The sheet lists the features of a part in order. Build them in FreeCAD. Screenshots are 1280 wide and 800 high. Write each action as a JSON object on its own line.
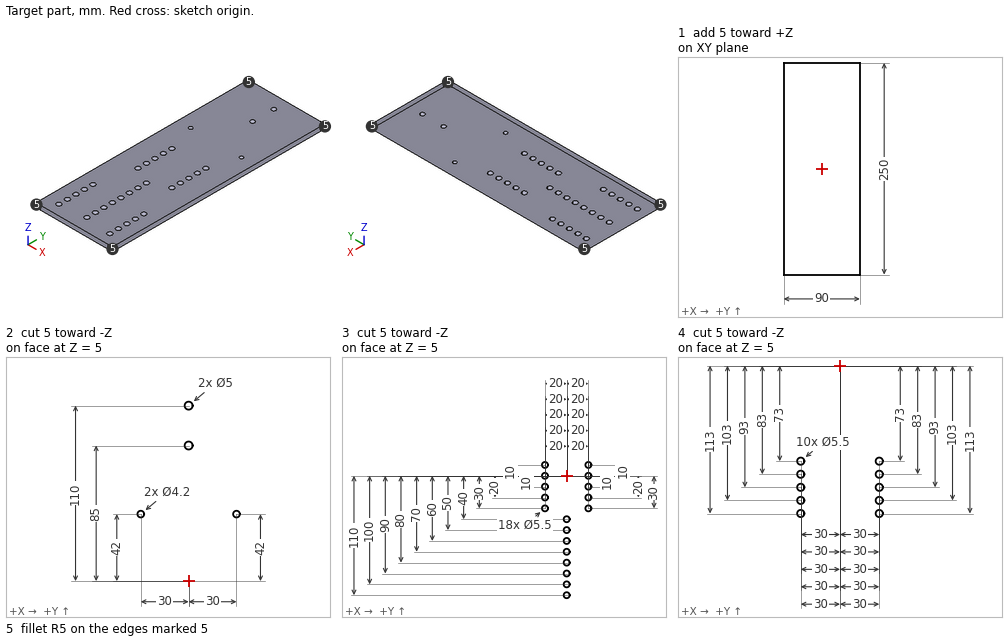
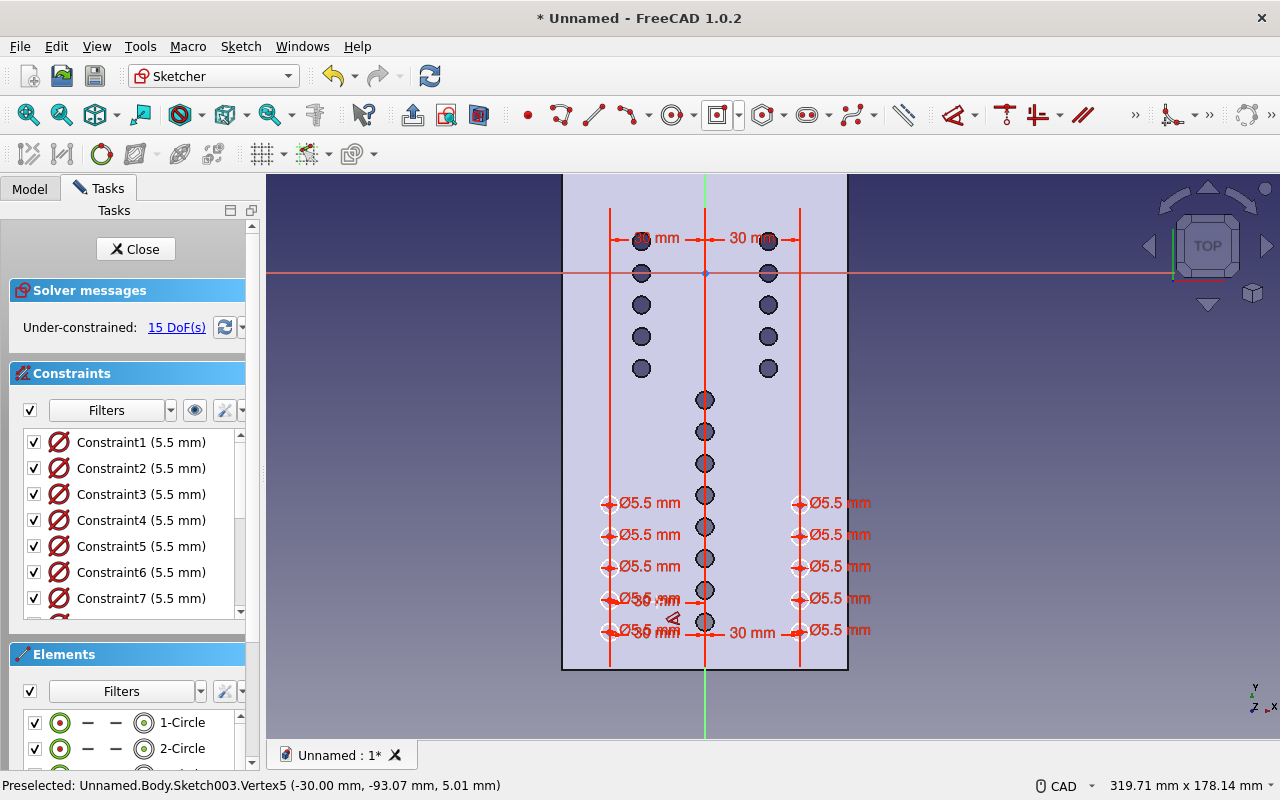
{"action": "left_click", "coordinate": [610, 568]}
{"action": "left_click", "coordinate": [576, 421]}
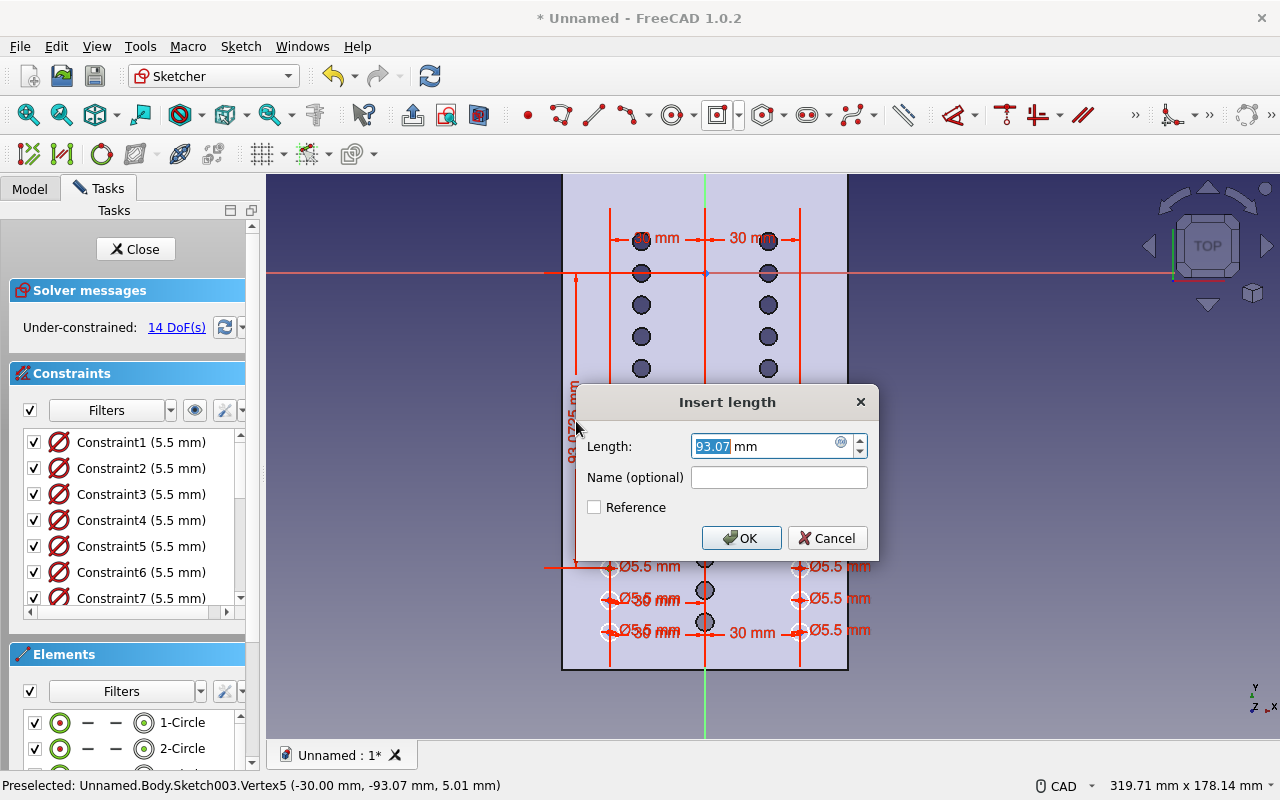
{"action": "type", "text": "93"}
{"action": "key", "text": "Return"}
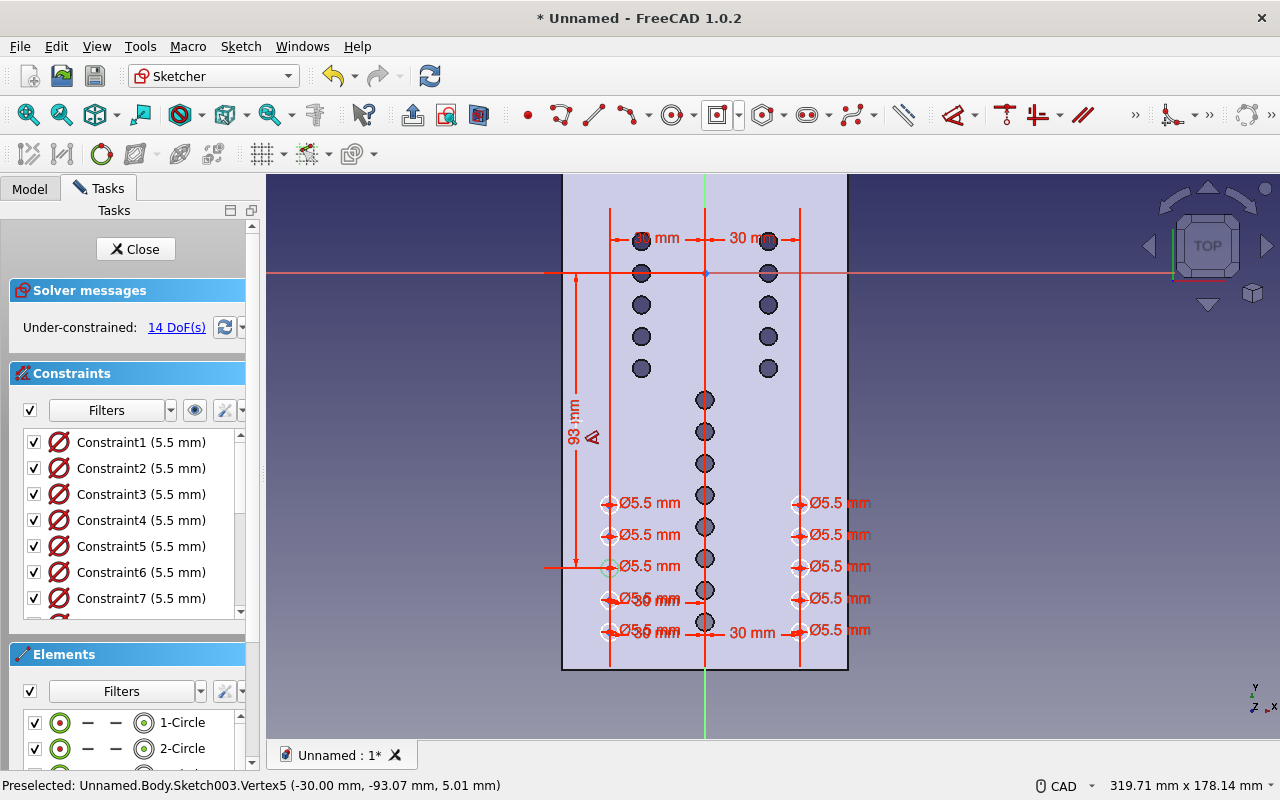
{"action": "left_click", "coordinate": [800, 568]}
{"action": "left_click", "coordinate": [753, 602]}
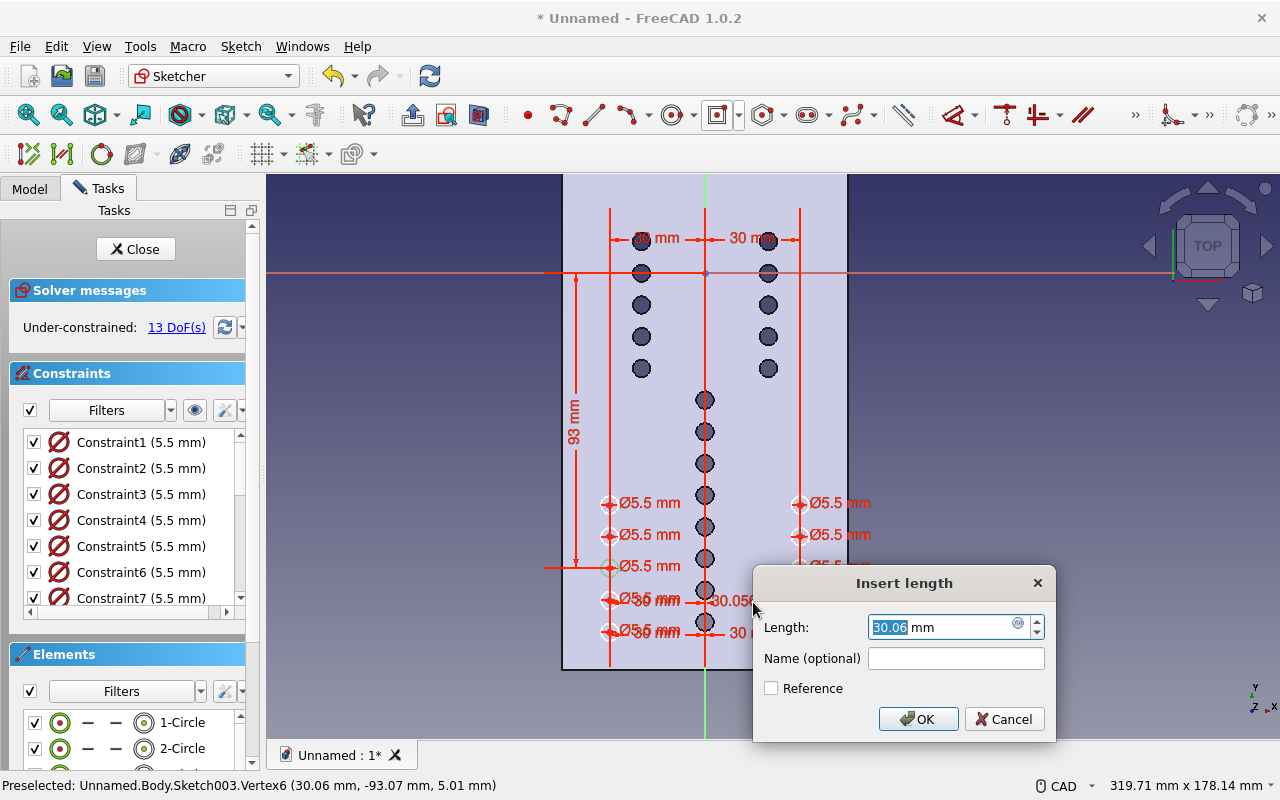
{"action": "type", "text": "30"}
{"action": "key", "text": "Return"}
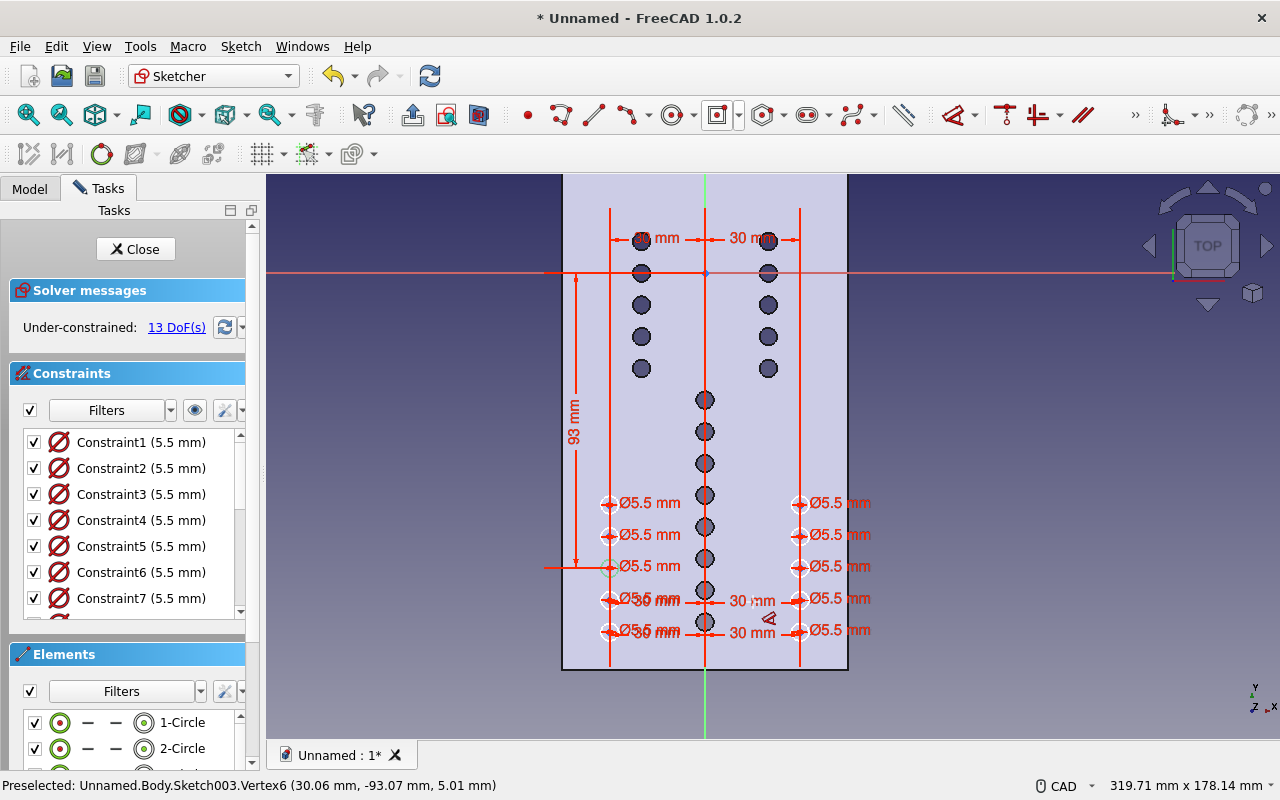
{"action": "left_click", "coordinate": [800, 568]}
{"action": "left_click", "coordinate": [834, 421]}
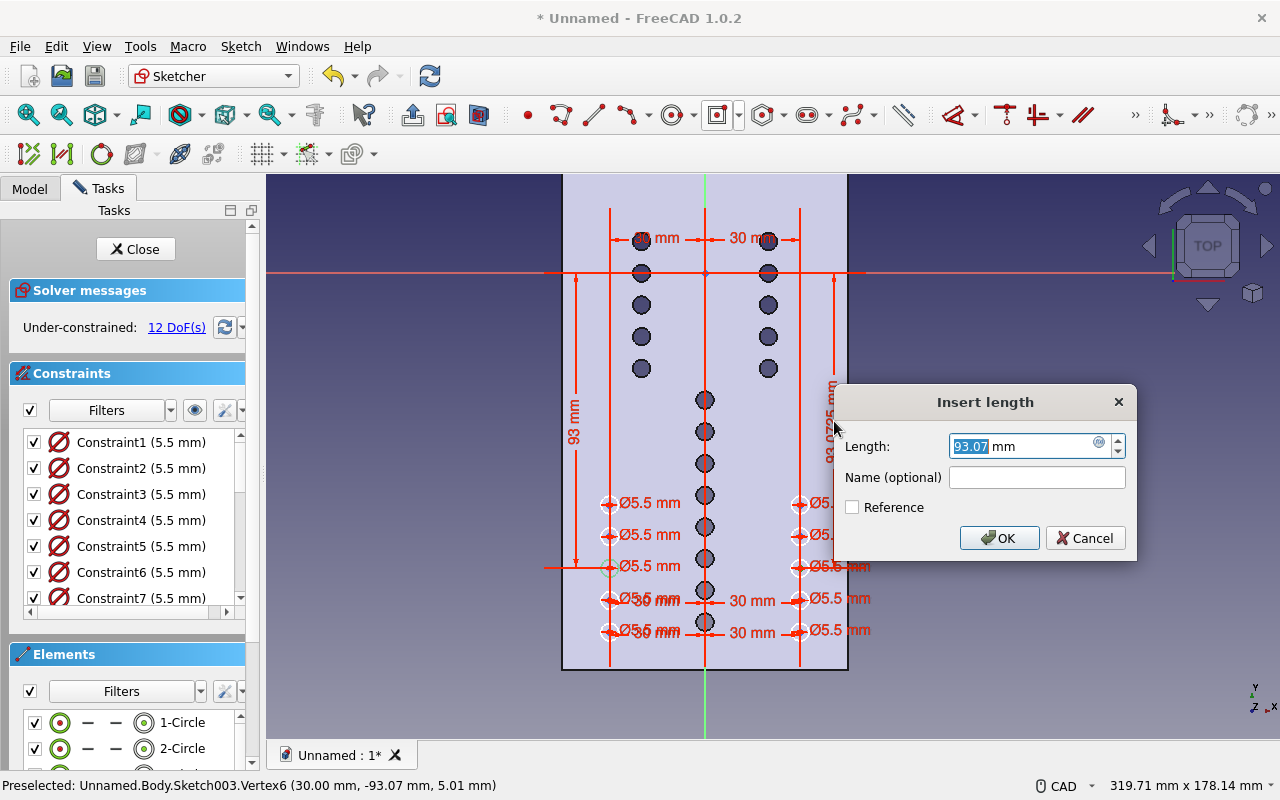
{"action": "type", "text": "93"}
{"action": "key", "text": "Return"}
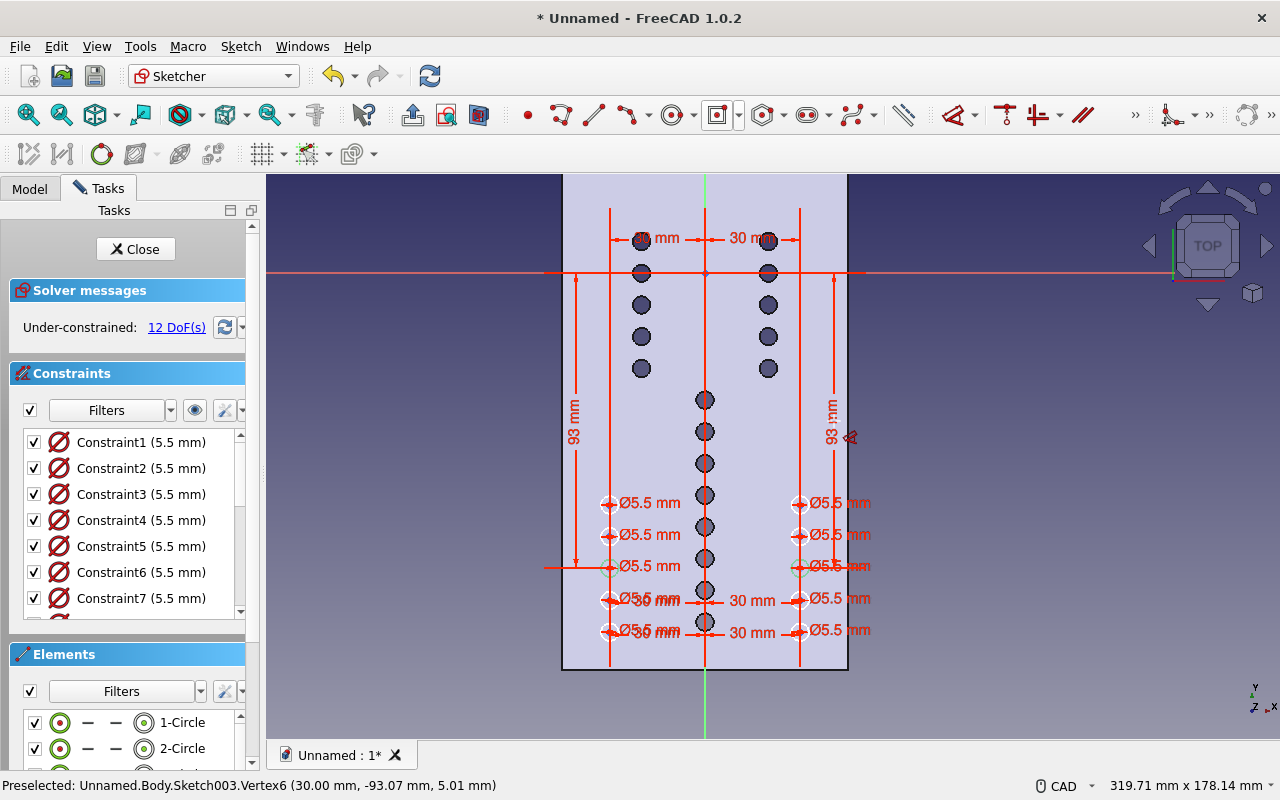
{"action": "left_click", "coordinate": [610, 537]}
{"action": "left_click", "coordinate": [657, 571]}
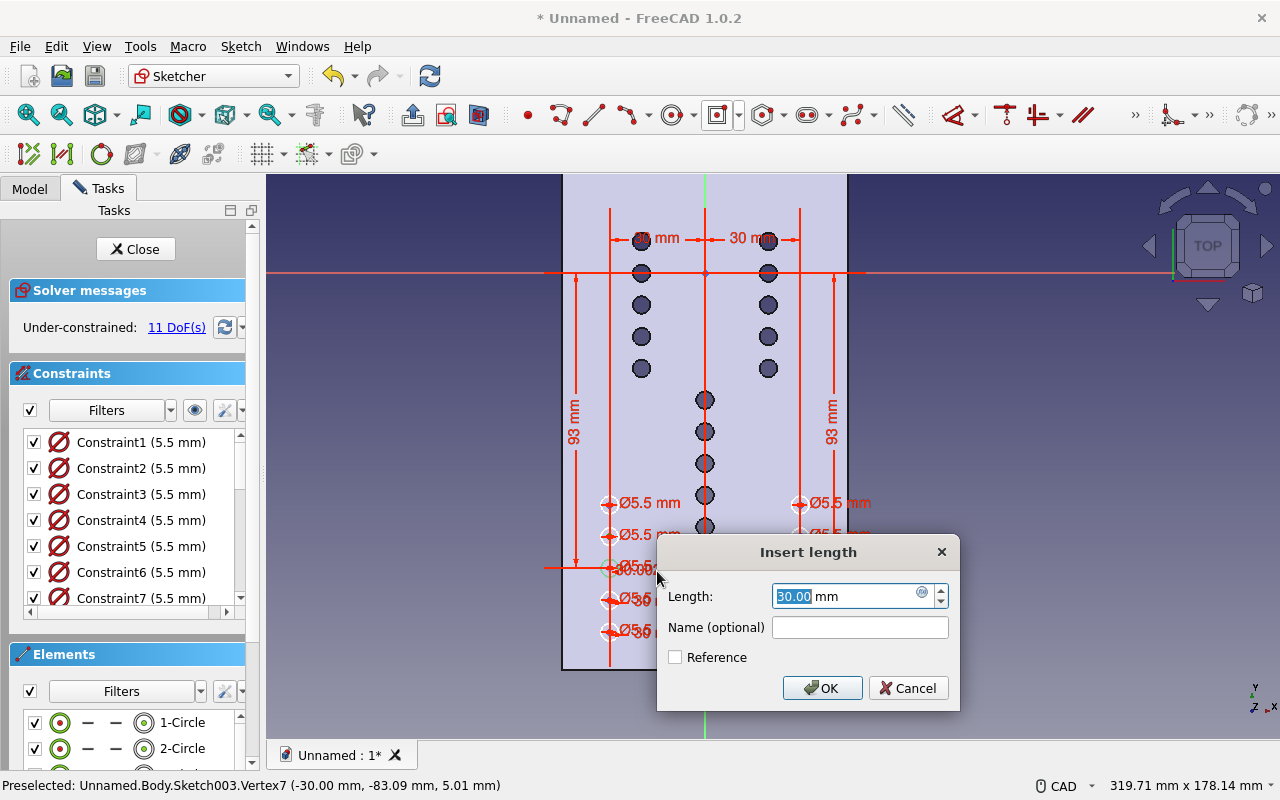
{"action": "type", "text": "30"}
{"action": "key", "text": "Return"}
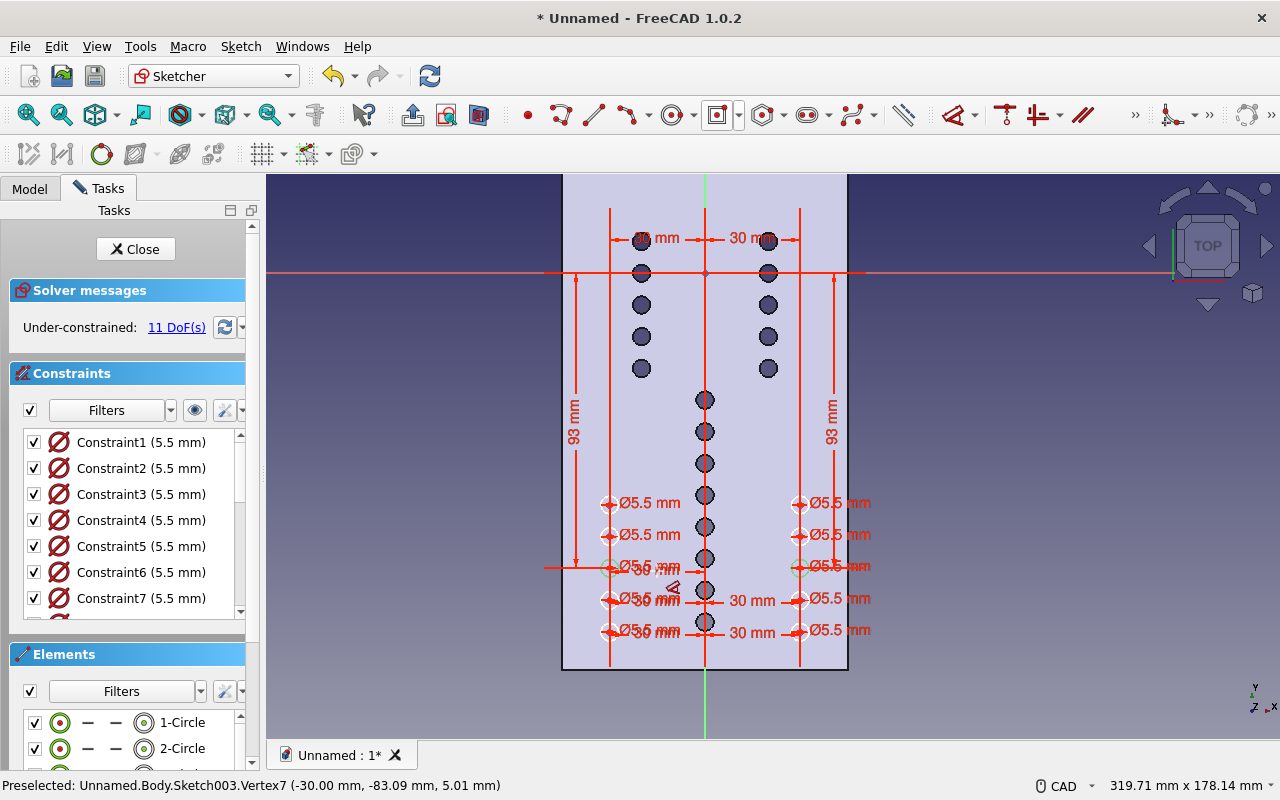
{"action": "left_click", "coordinate": [610, 537]}
{"action": "left_click", "coordinate": [576, 344]}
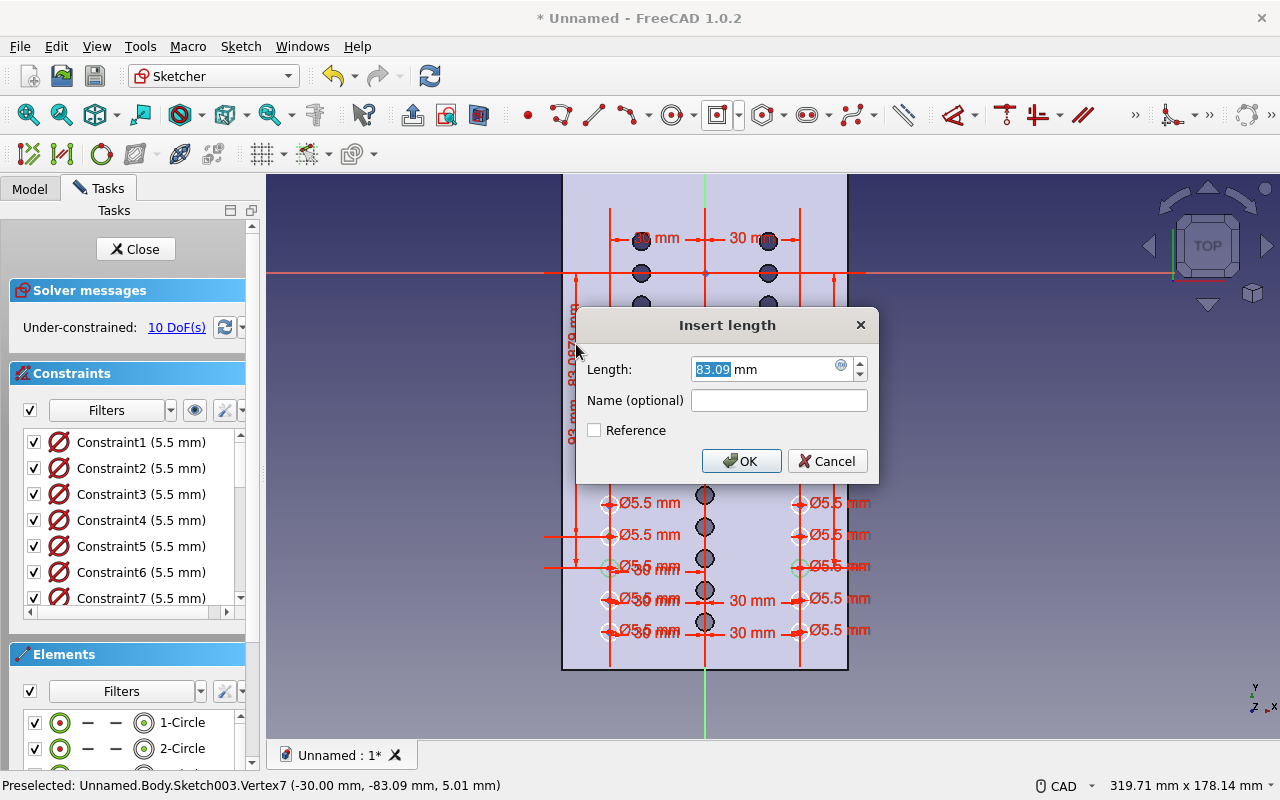
{"action": "type", "text": "83"}
{"action": "key", "text": "Return"}